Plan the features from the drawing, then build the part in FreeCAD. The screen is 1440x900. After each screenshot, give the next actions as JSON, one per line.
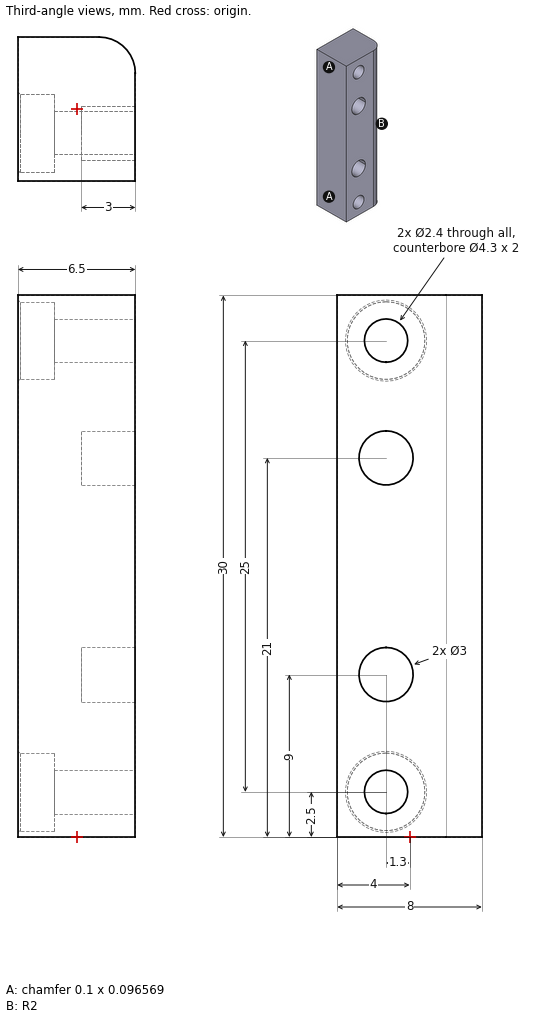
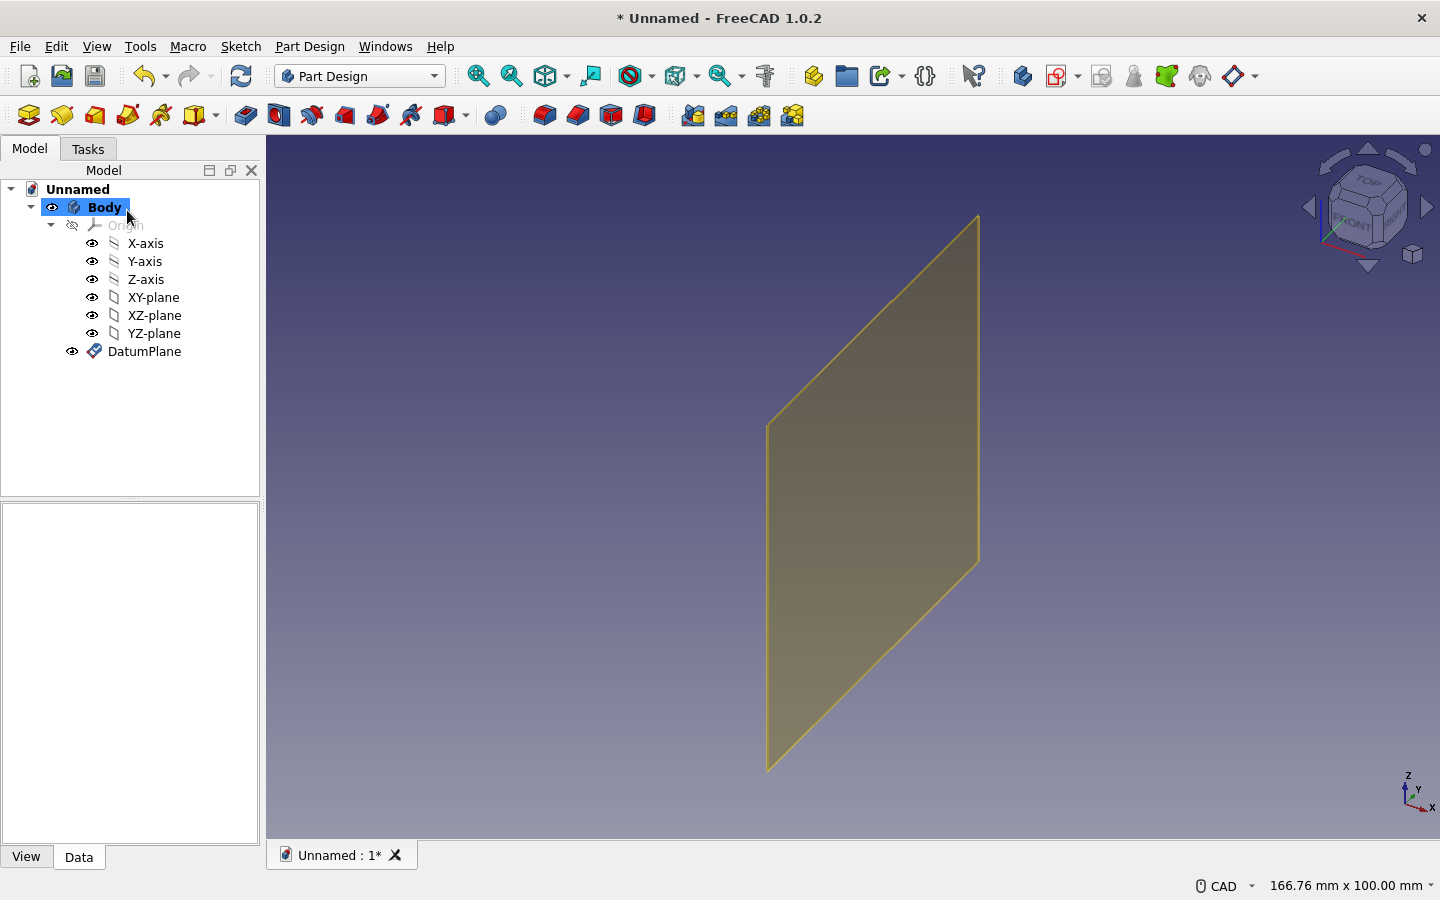
{"action": "left_click", "coordinate": [117, 351]}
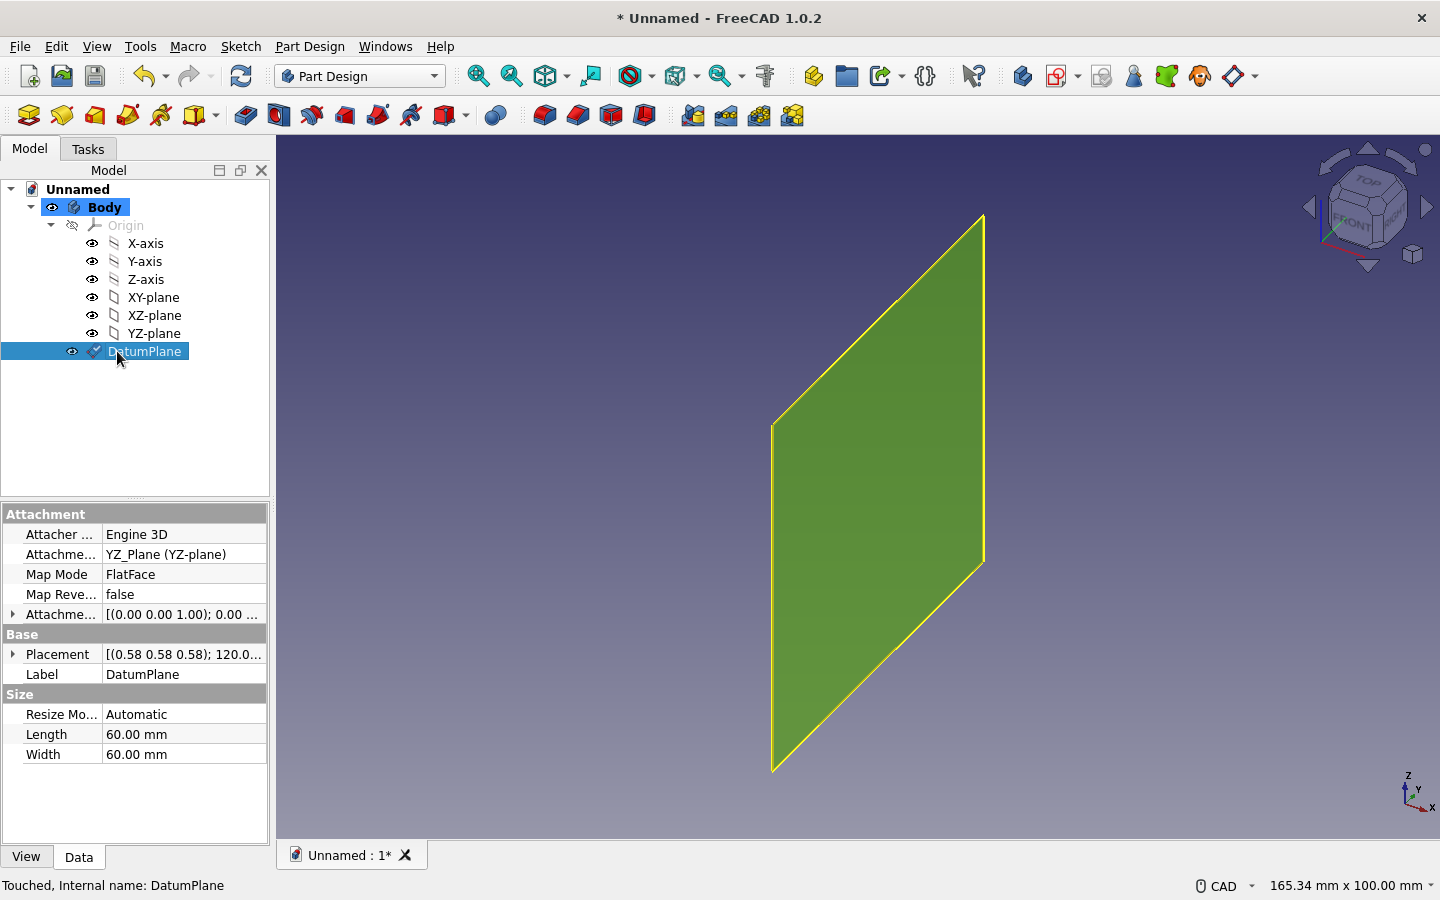
{"action": "left_click", "coordinate": [1056, 76]}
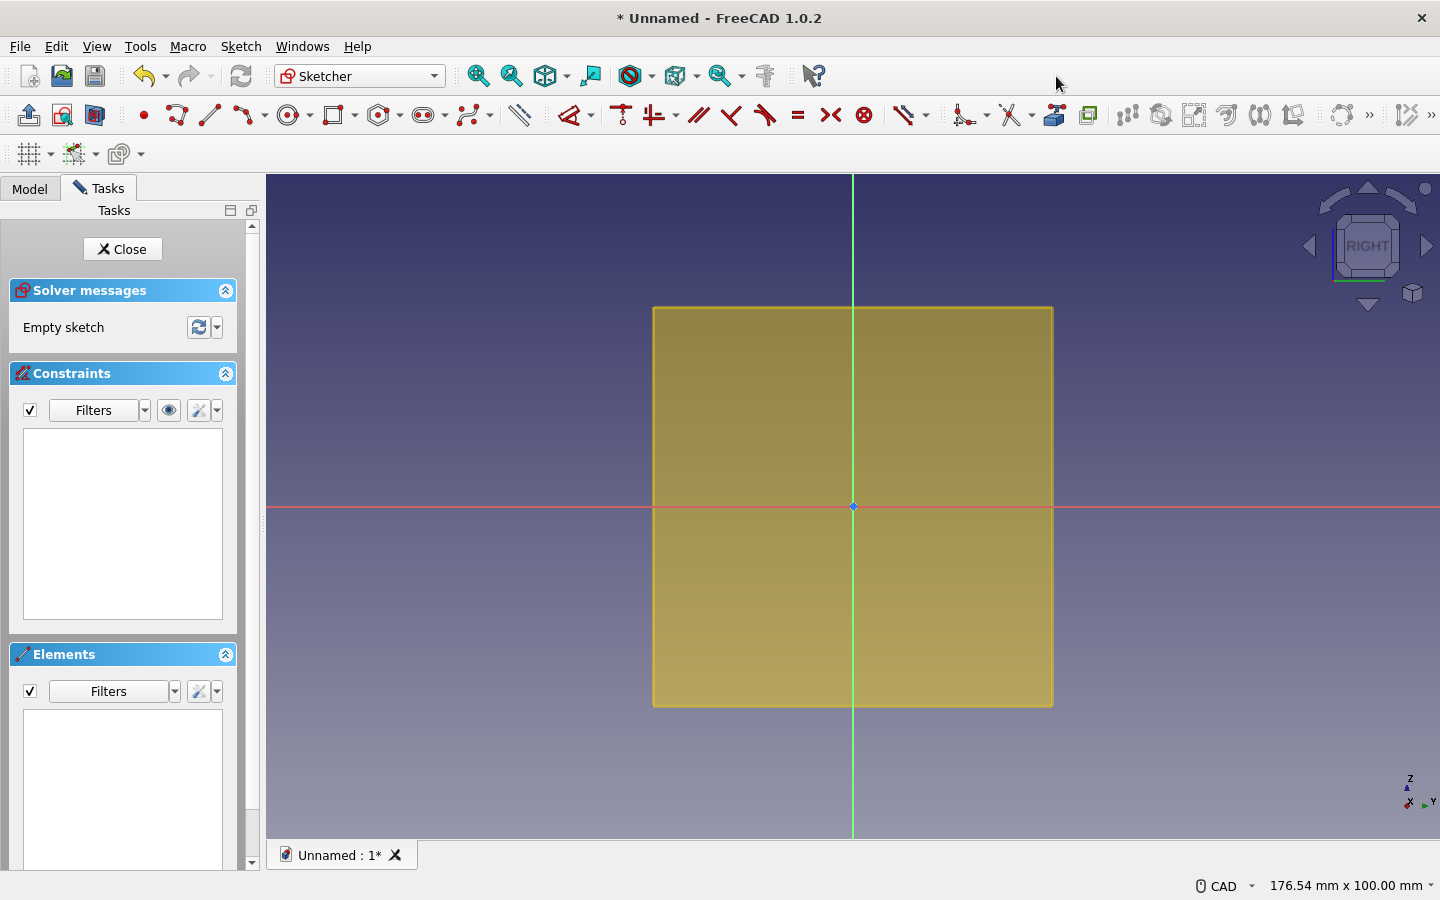
{"action": "scroll", "coordinate": [909, 325], "scroll_direction": "up", "scroll_amount": 4}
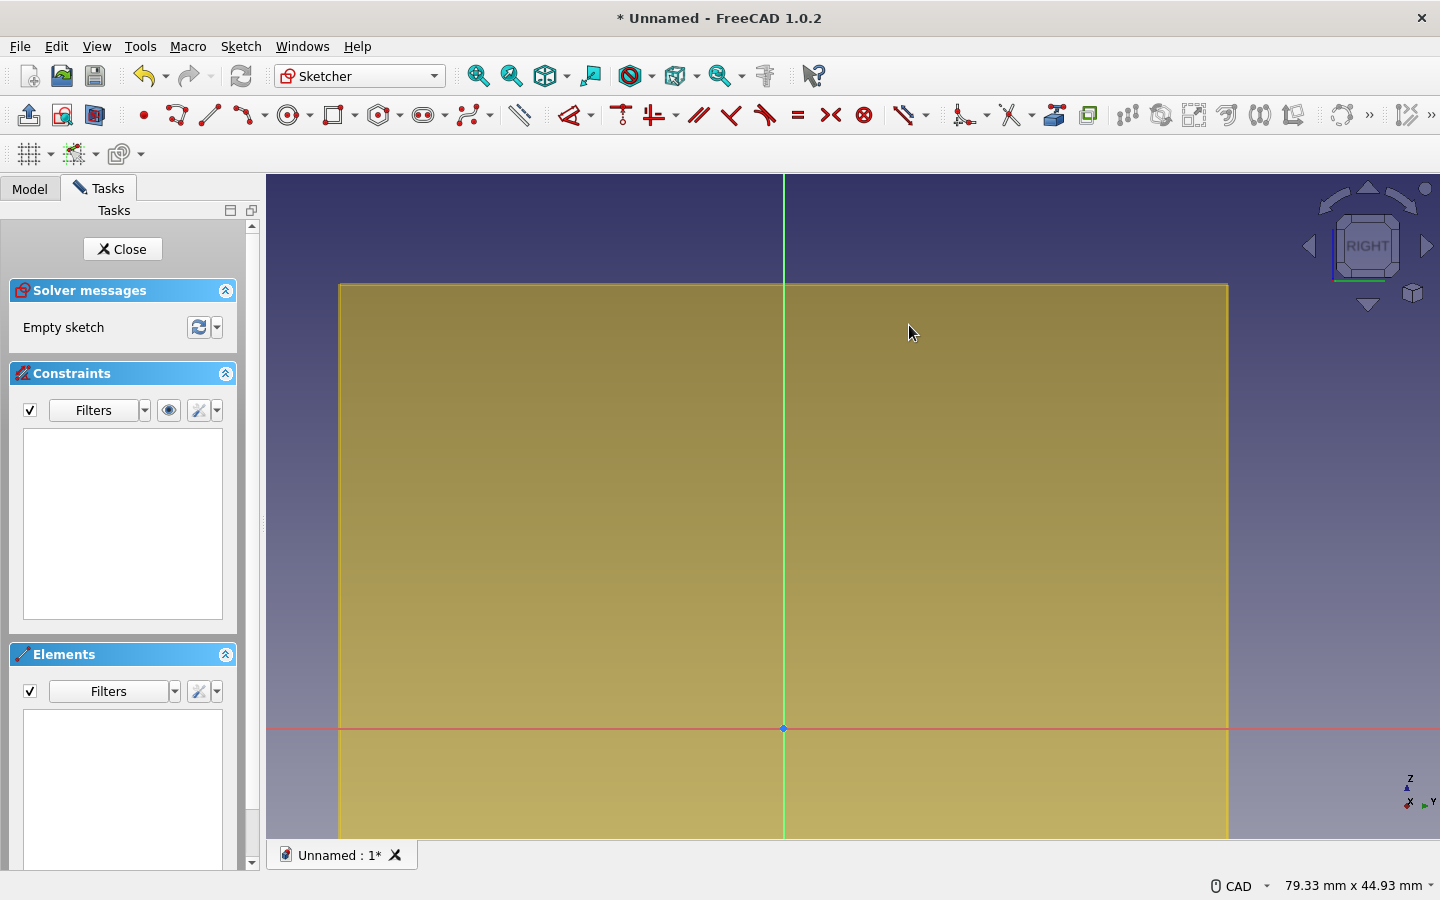
{"action": "left_click", "coordinate": [332, 116]}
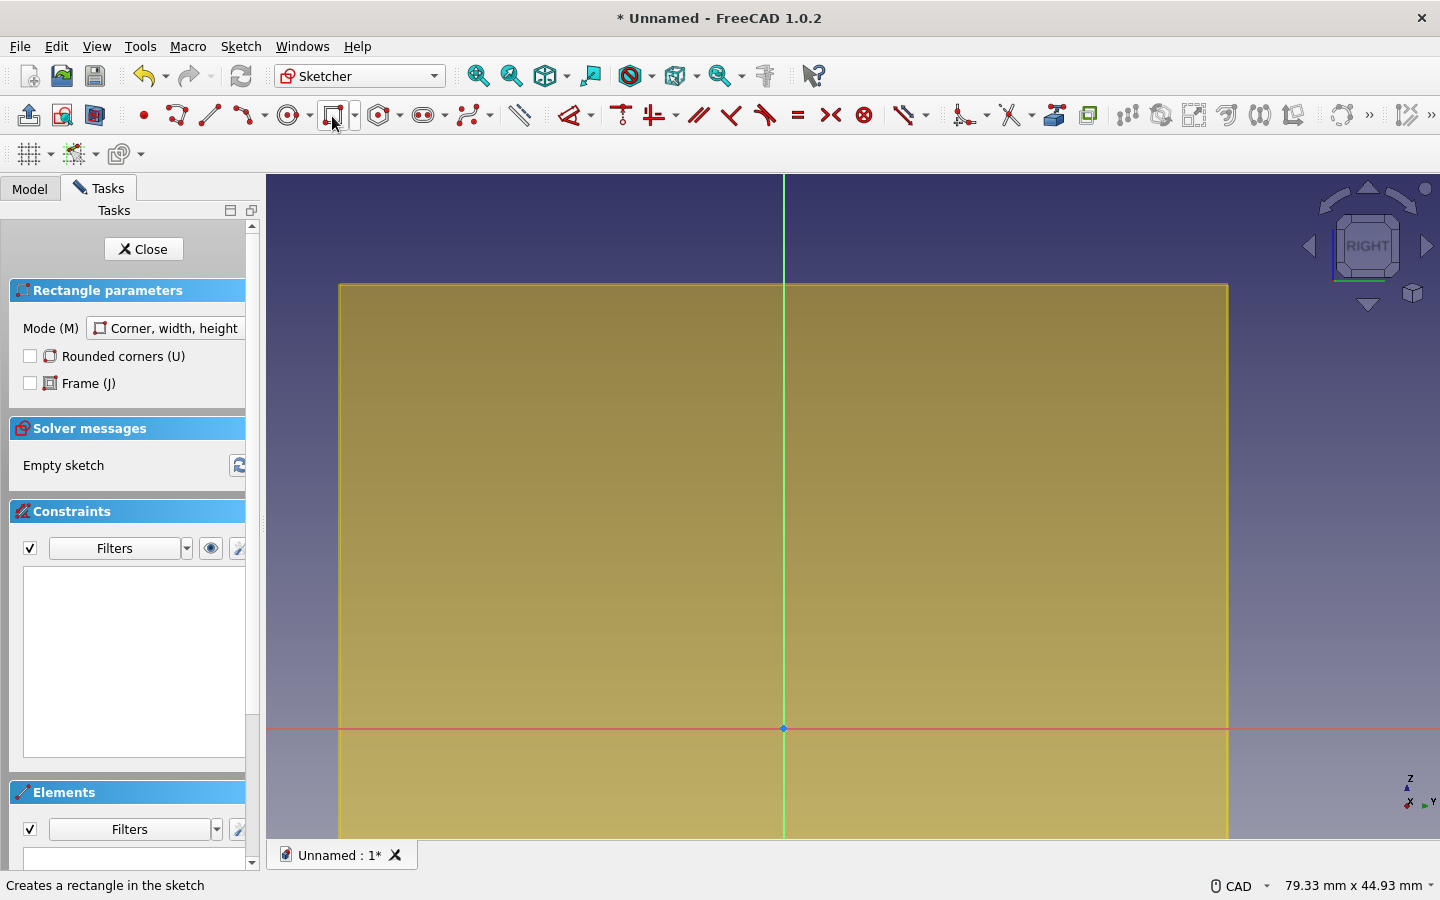
{"action": "left_click", "coordinate": [724, 285]}
{"action": "left_click", "coordinate": [843, 729]}
{"action": "key", "text": "Escape"}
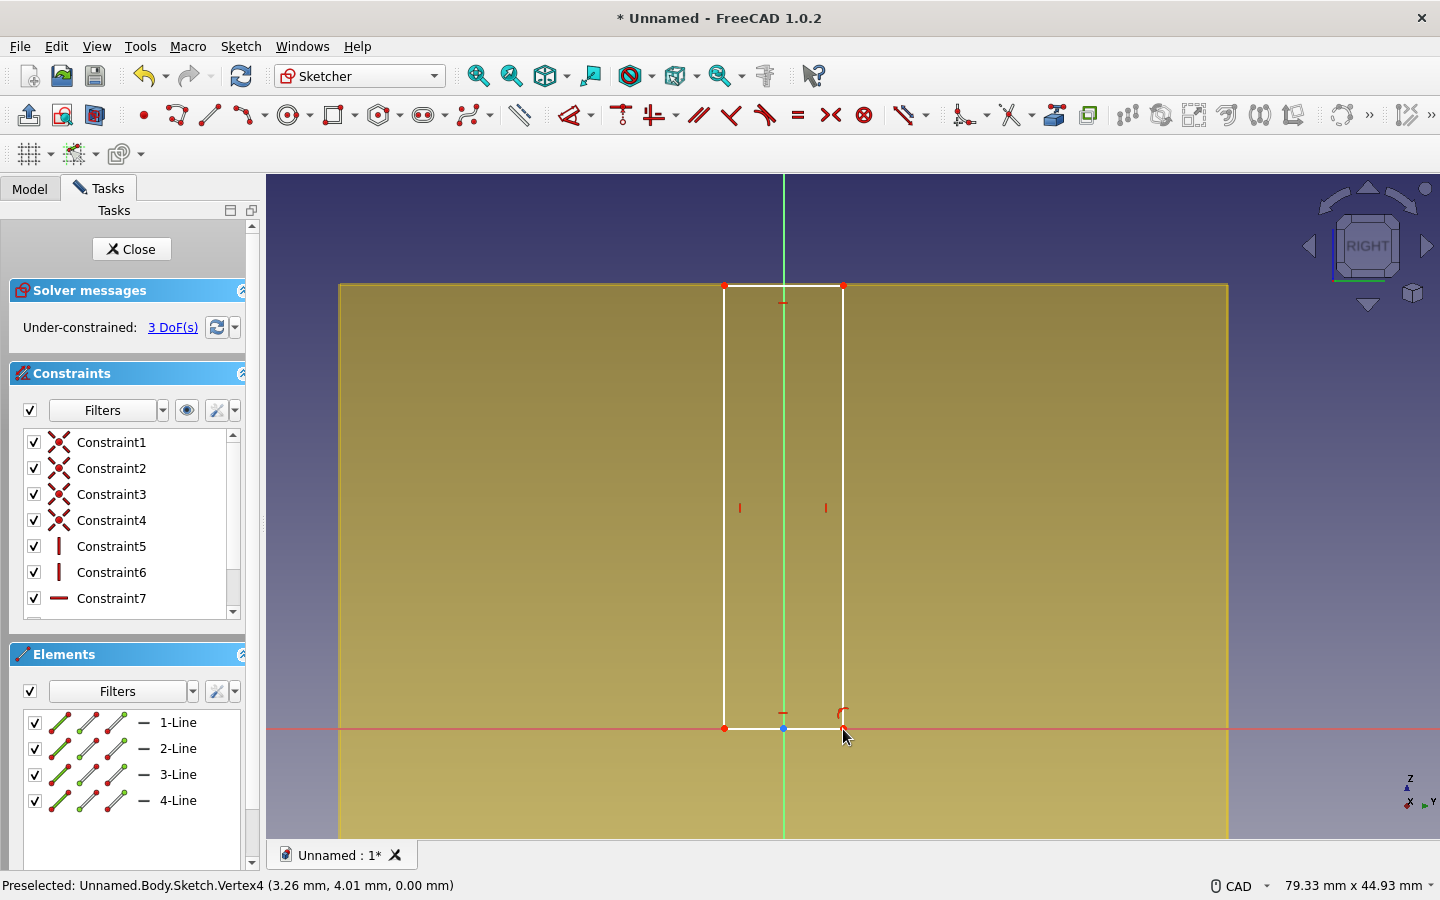
{"action": "left_click", "coordinate": [760, 729]}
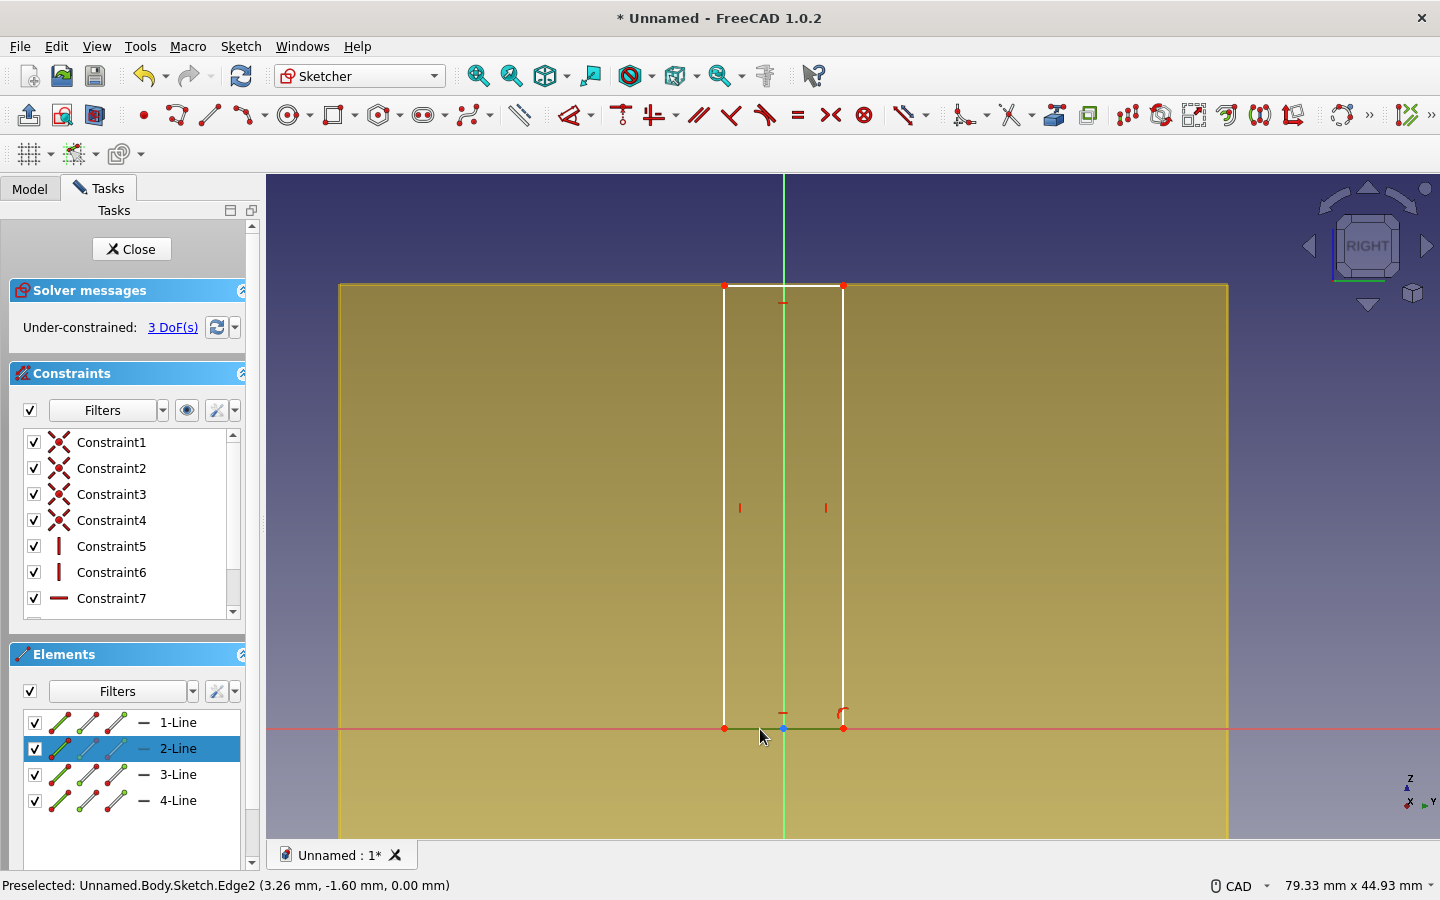
{"action": "left_click", "coordinate": [590, 116]}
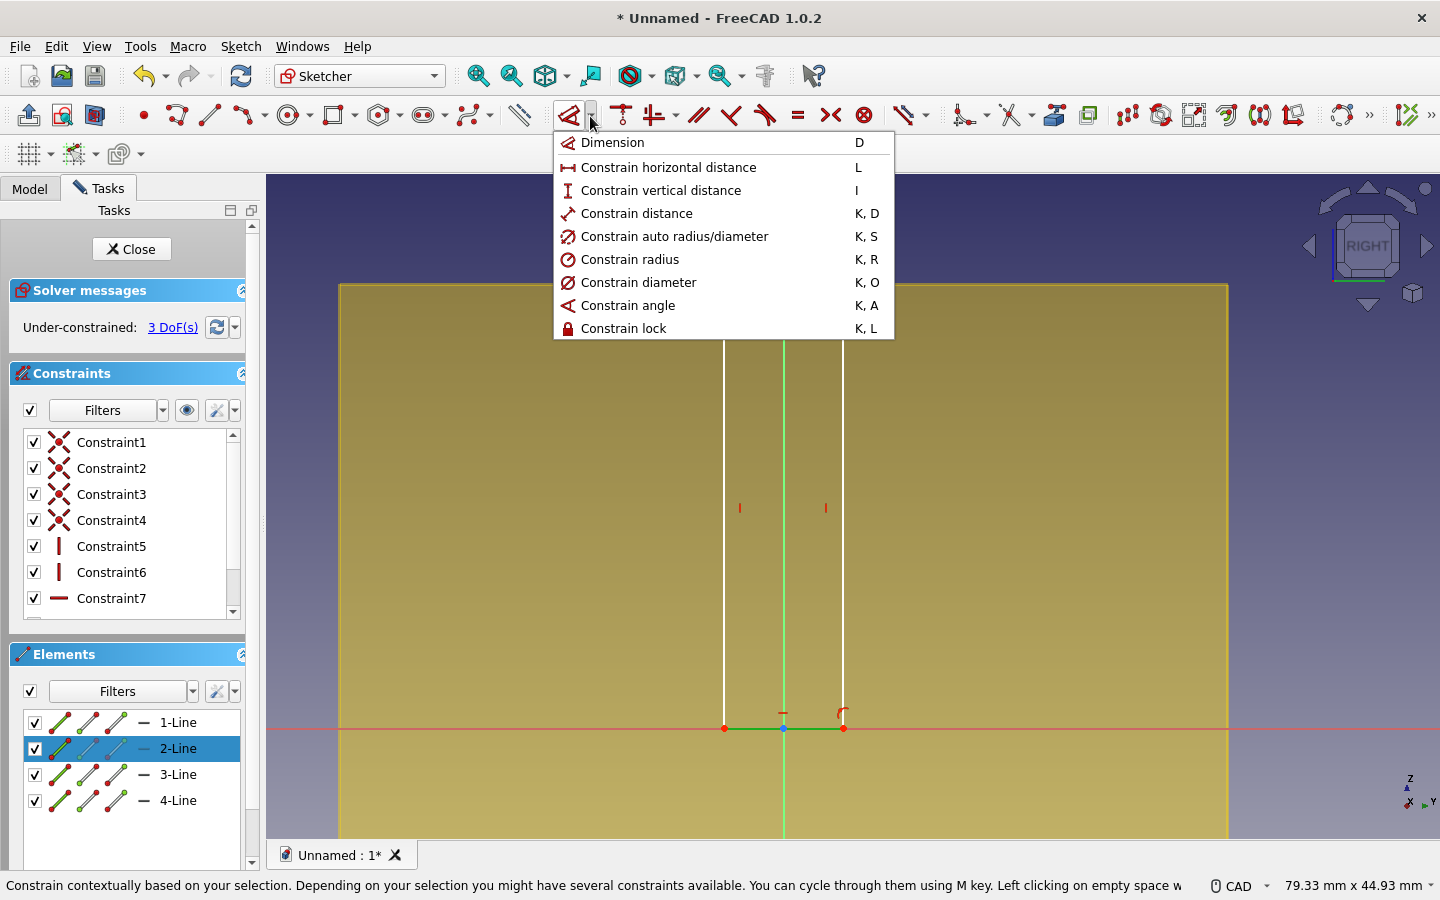
{"action": "left_click", "coordinate": [724, 168]}